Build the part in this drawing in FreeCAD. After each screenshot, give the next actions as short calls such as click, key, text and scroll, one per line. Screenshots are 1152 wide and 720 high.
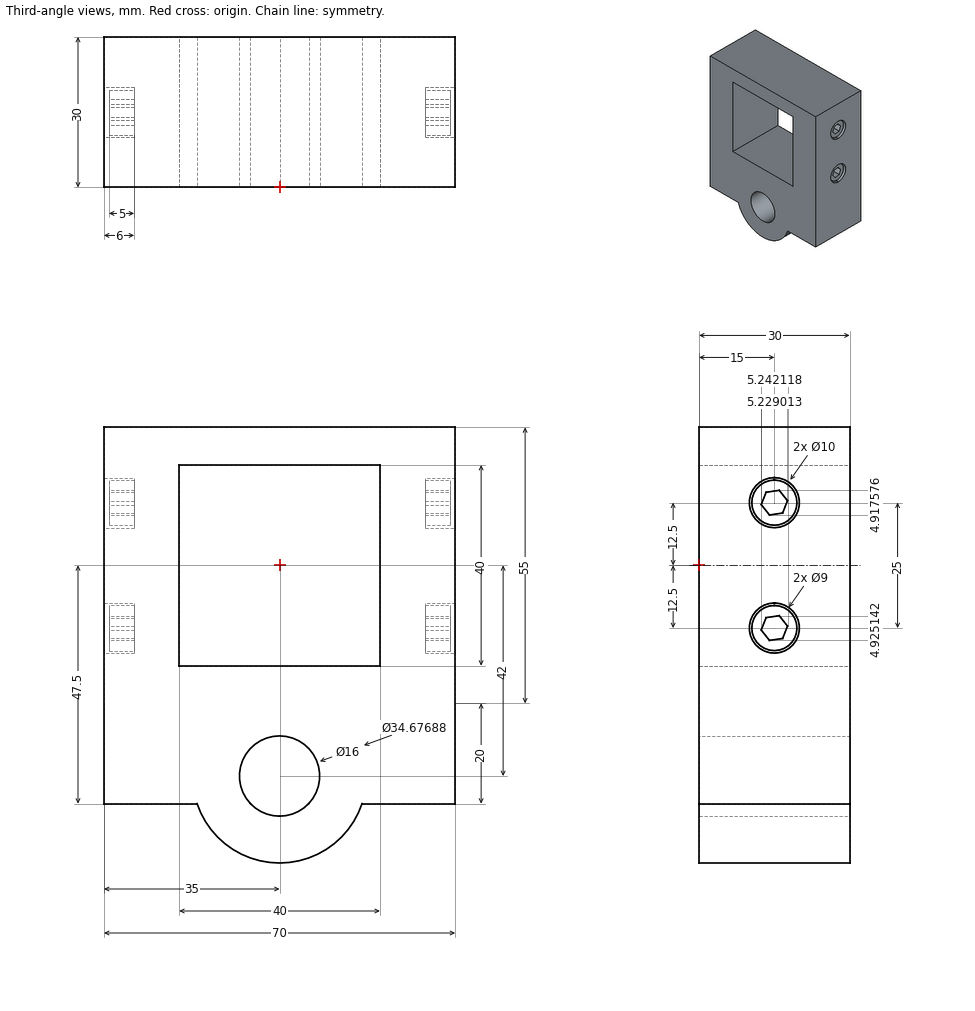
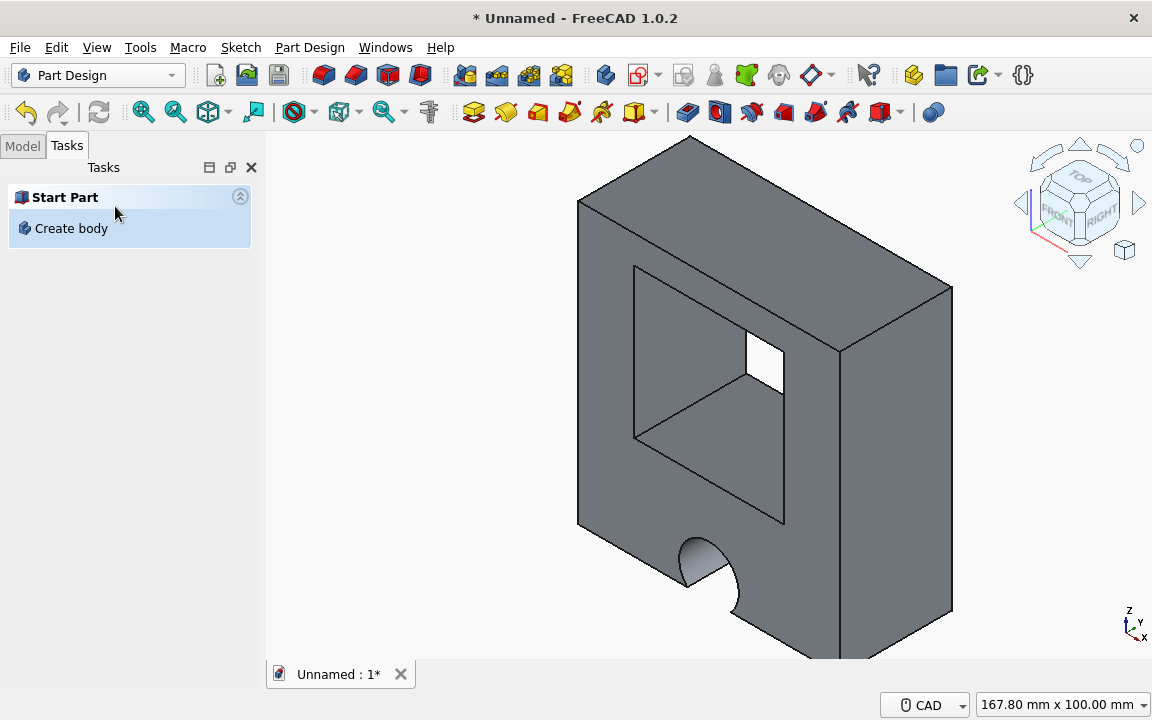
click(144, 112)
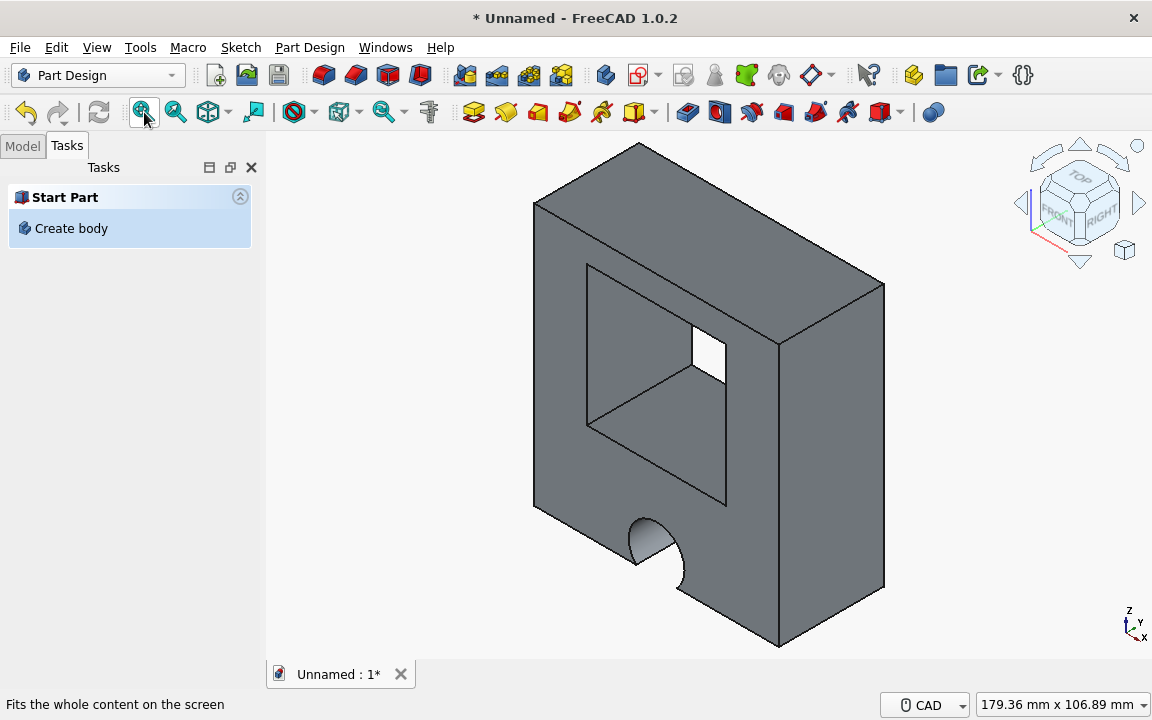
click(726, 551)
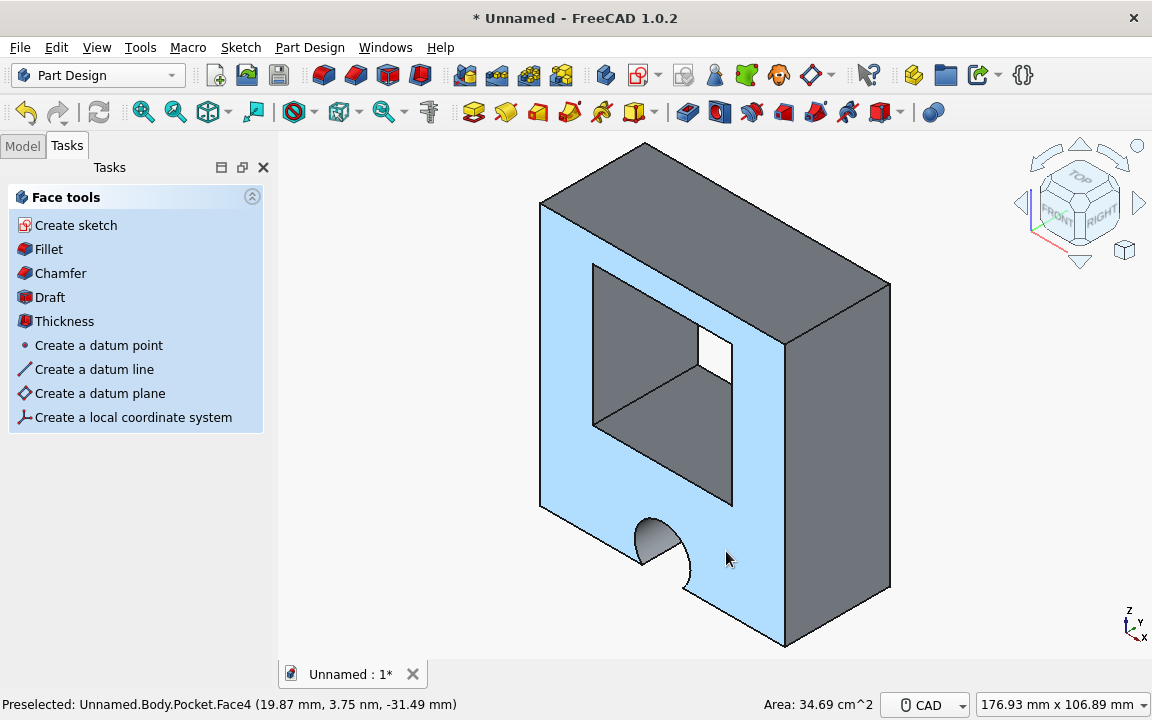
click(638, 76)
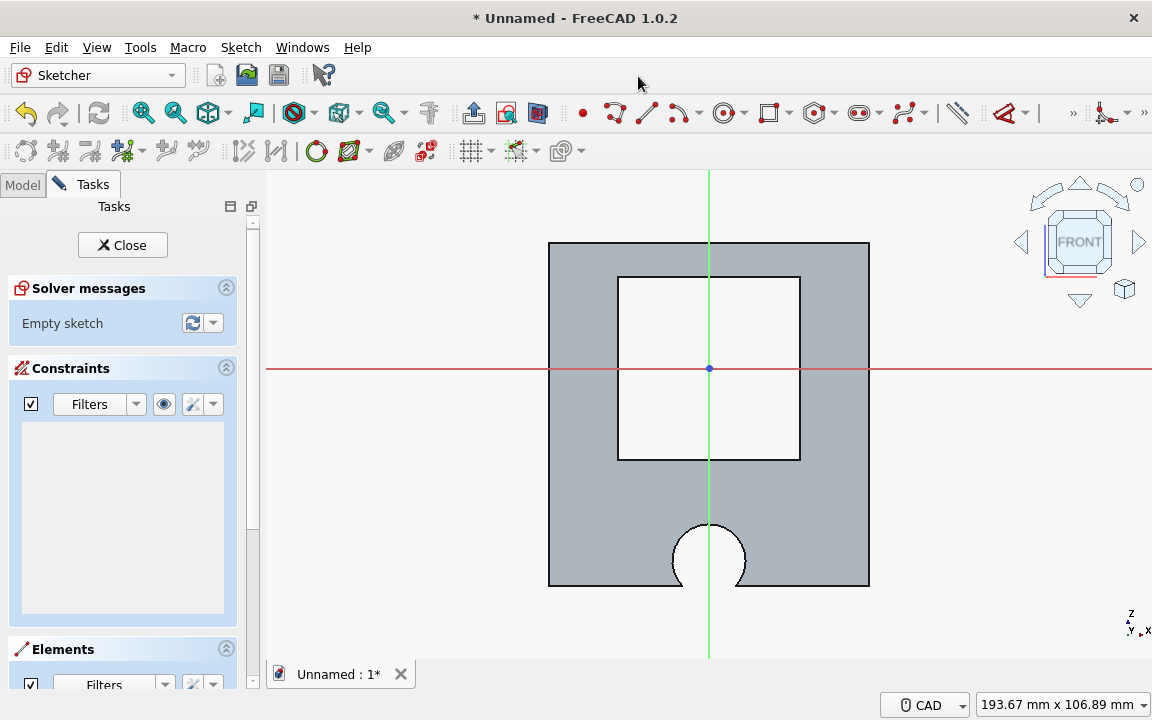
scroll(331, 198, down, 1)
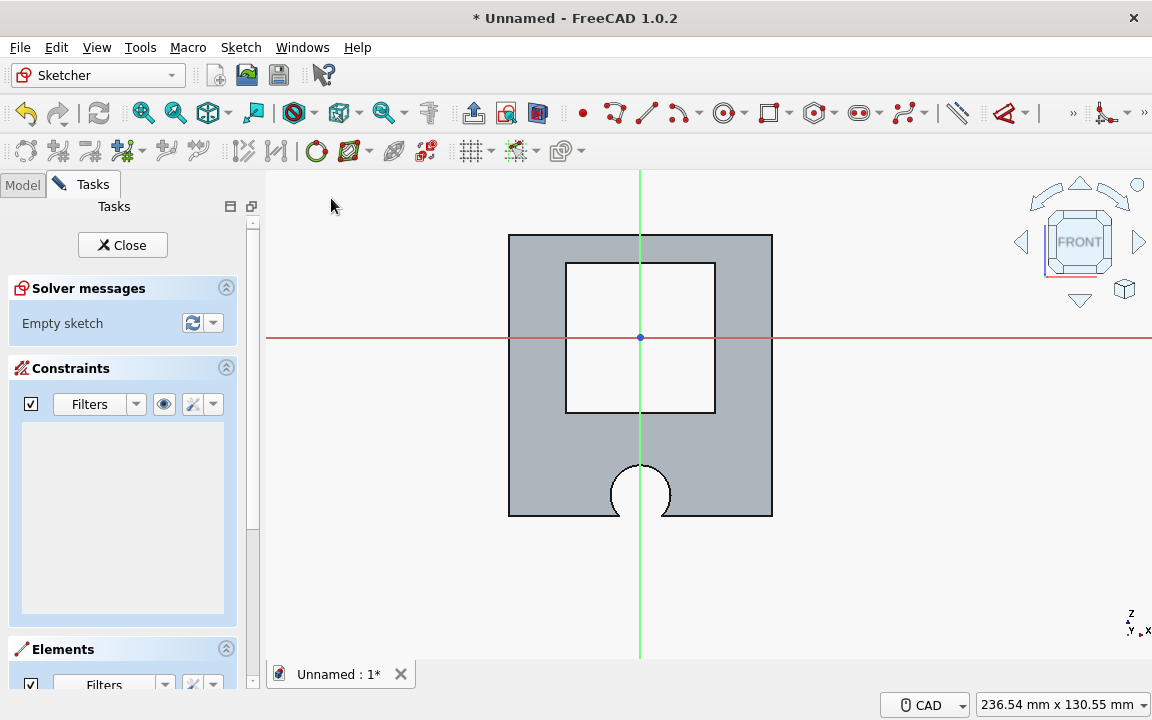
scroll(640, 519, up, 2)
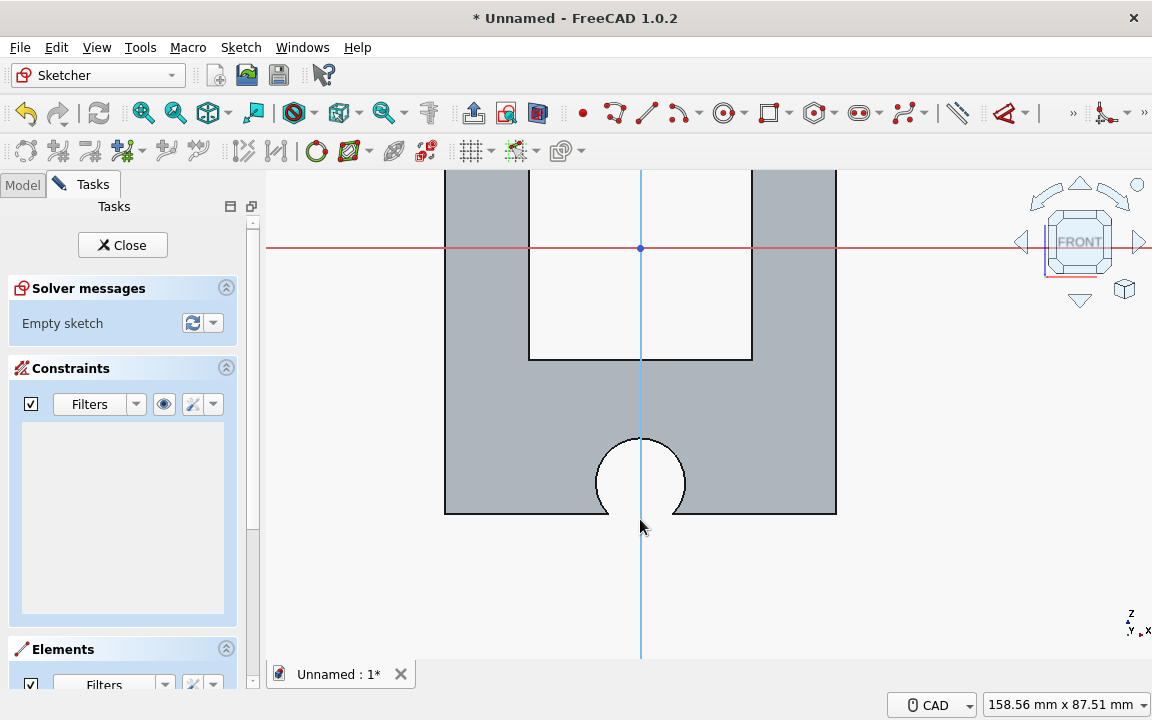
click(724, 114)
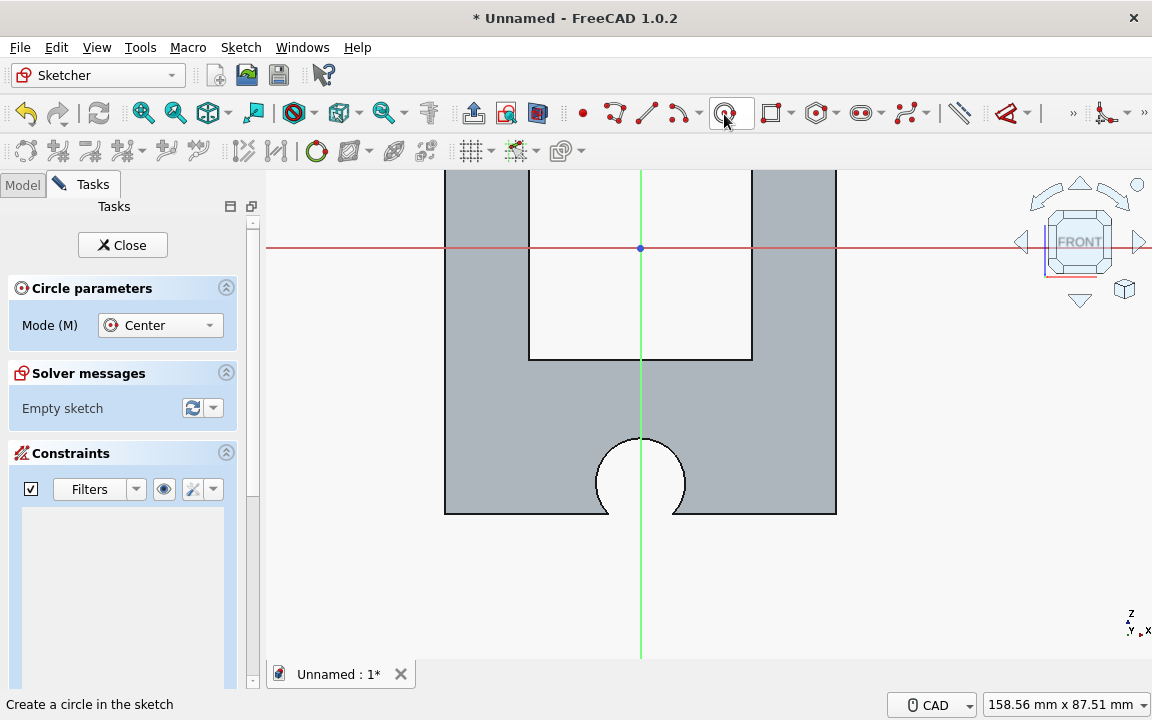
click(641, 483)
move(709, 415)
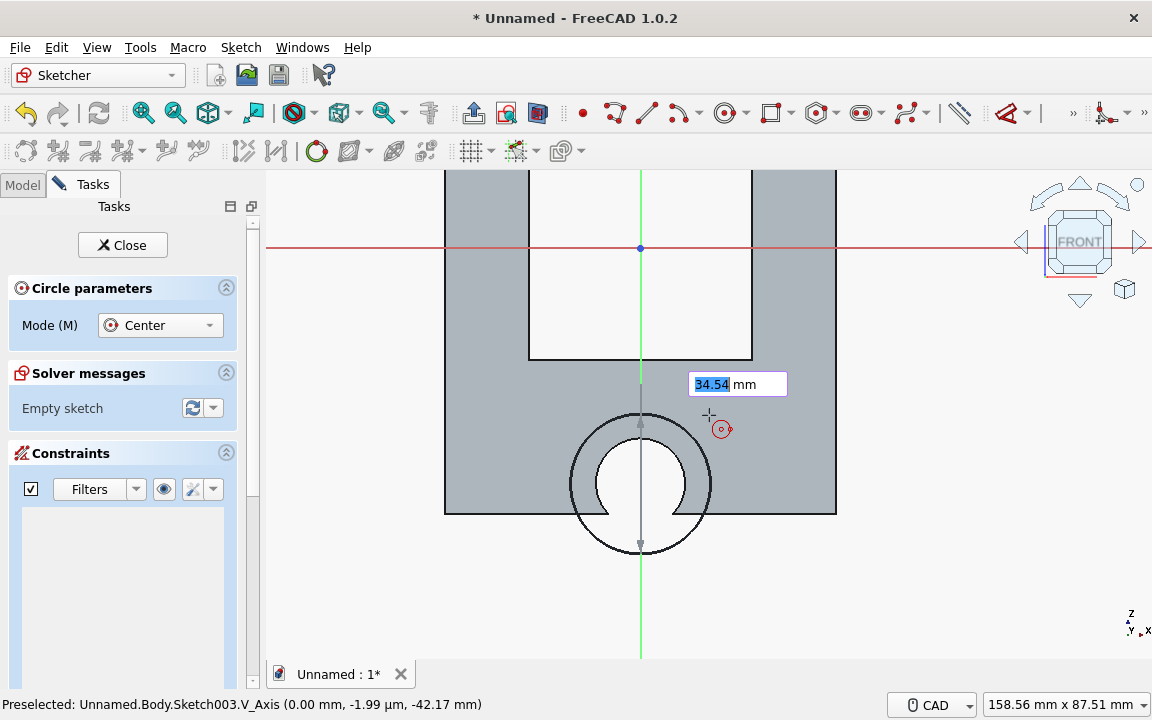
text(34.67688)
key(Return)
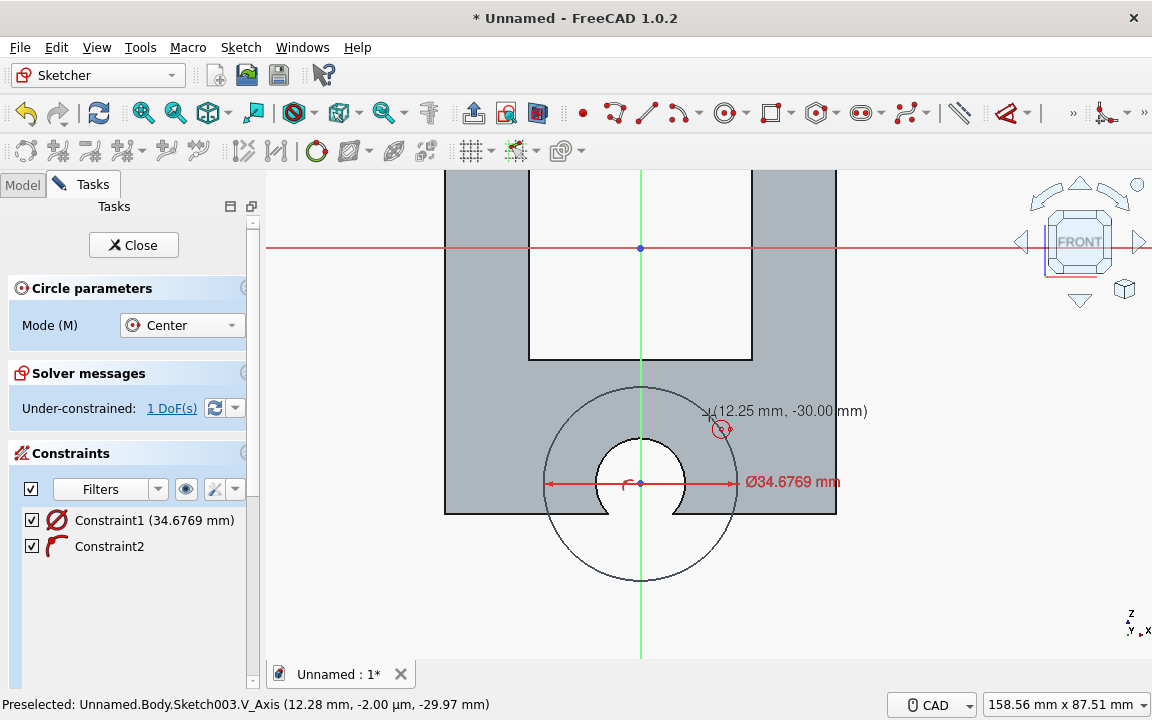
click(641, 484)
move(672, 451)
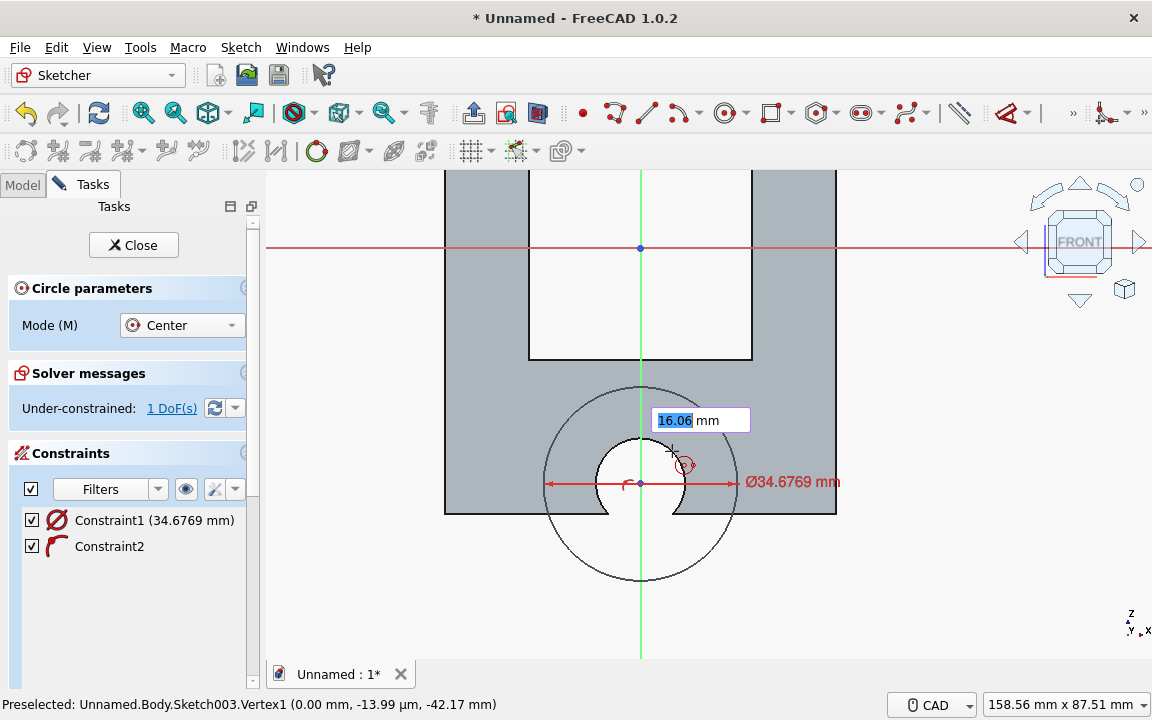
text(16)
key(Return)
key(Escape)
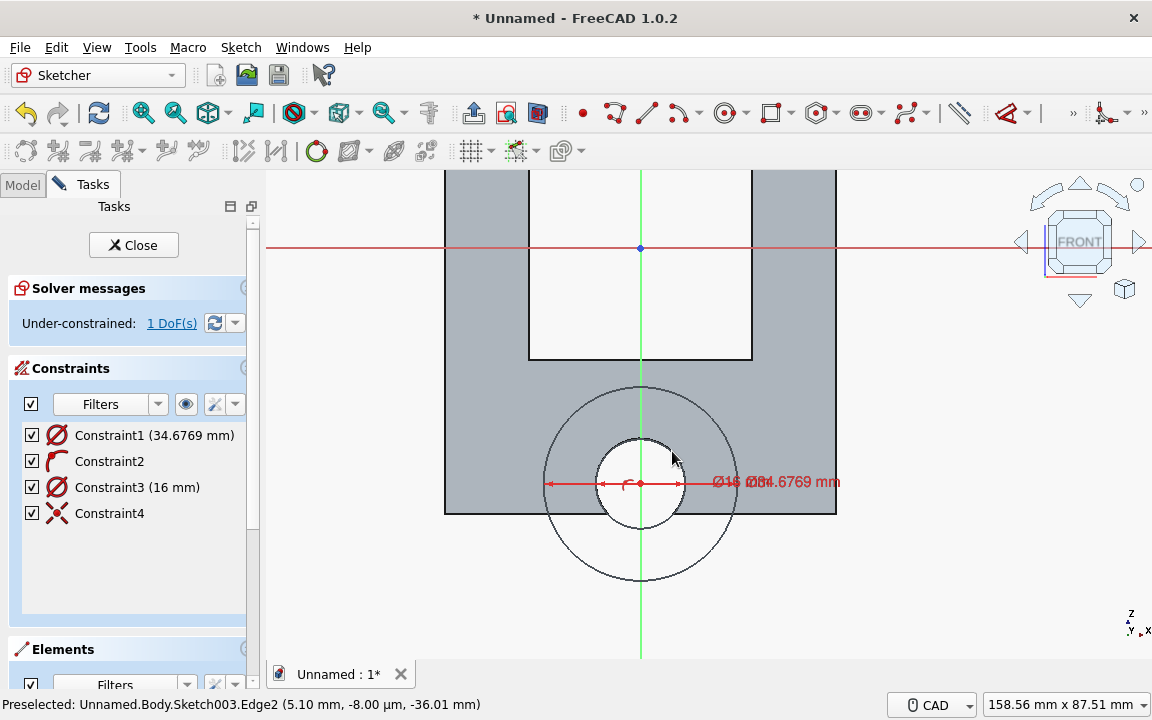
click(1006, 114)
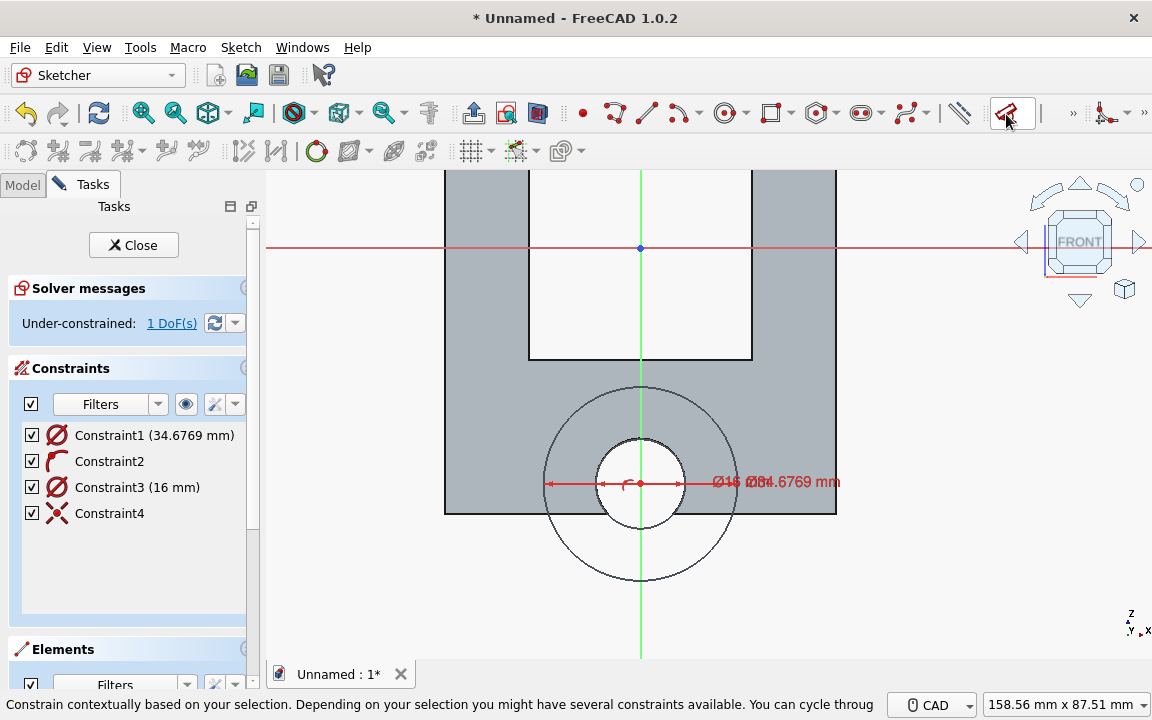
click(641, 484)
click(675, 366)